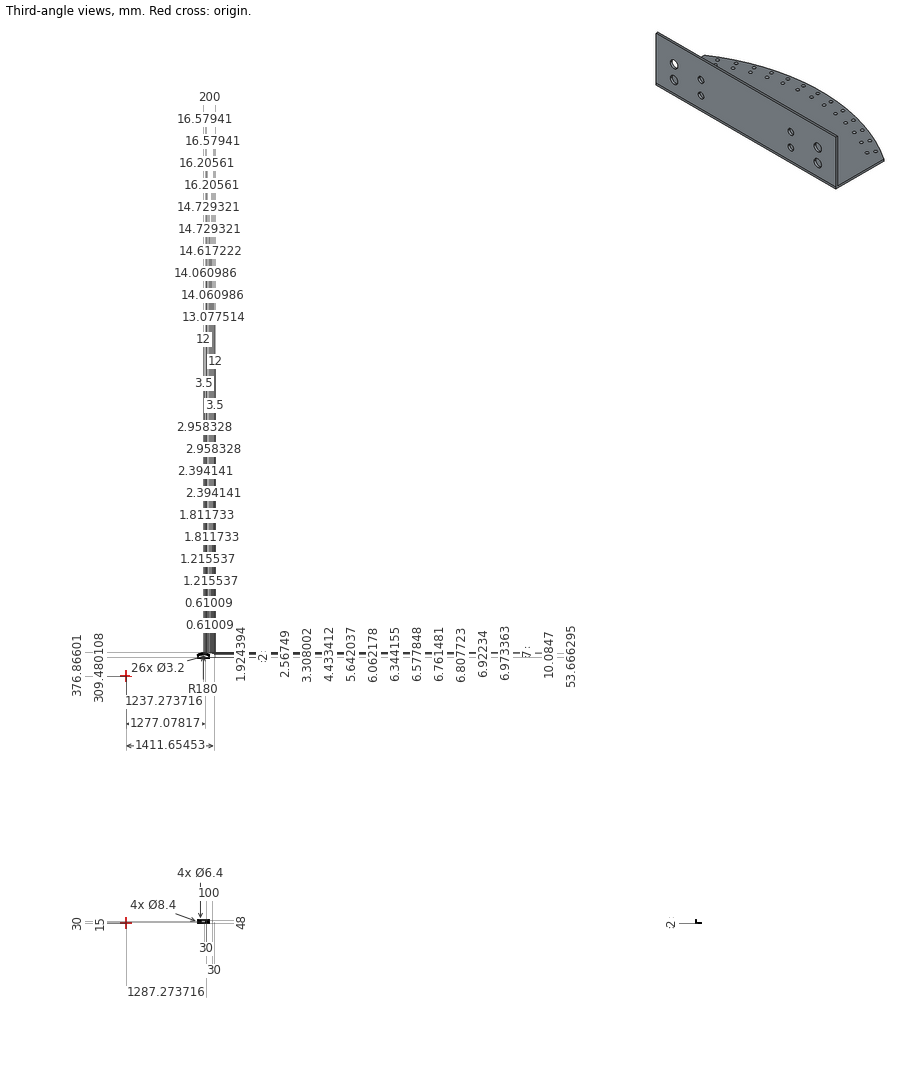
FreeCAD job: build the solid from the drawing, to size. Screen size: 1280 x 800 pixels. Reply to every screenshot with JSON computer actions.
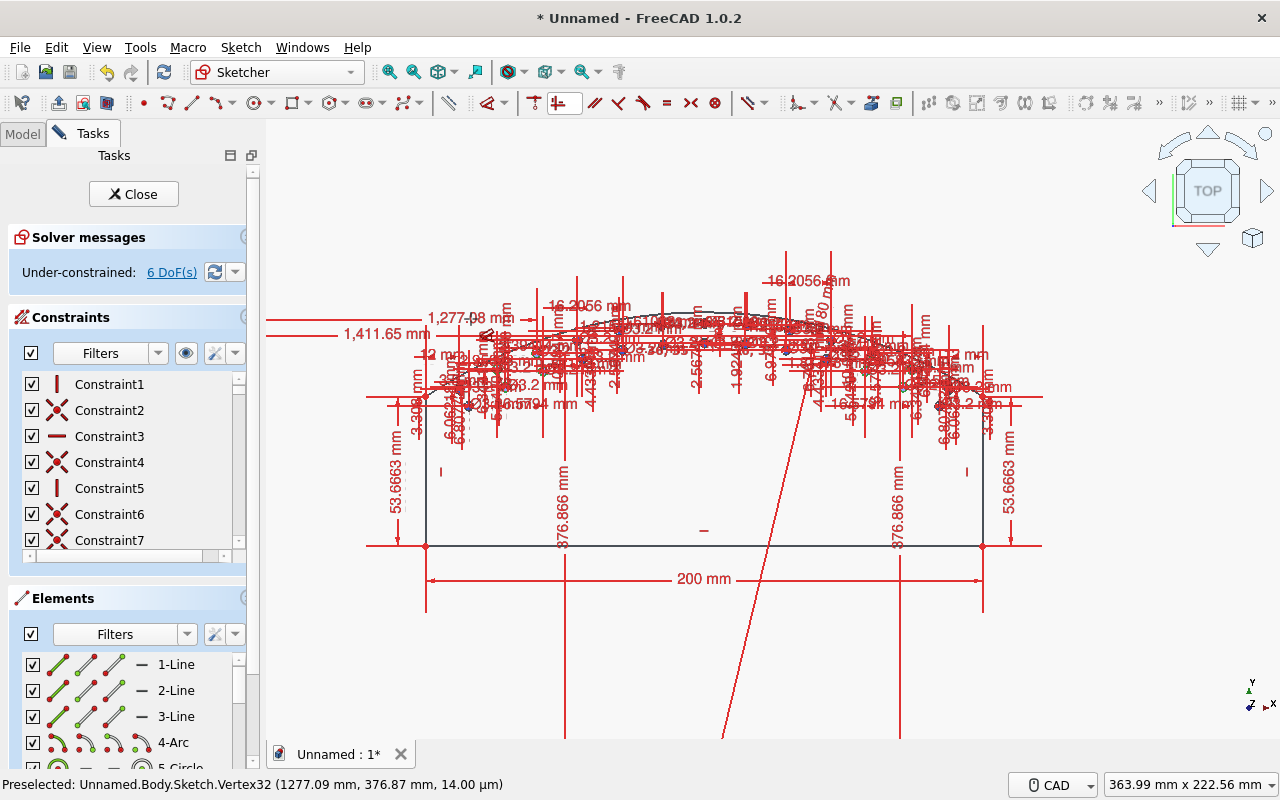
{"action": "left_click", "coordinate": [940, 406]}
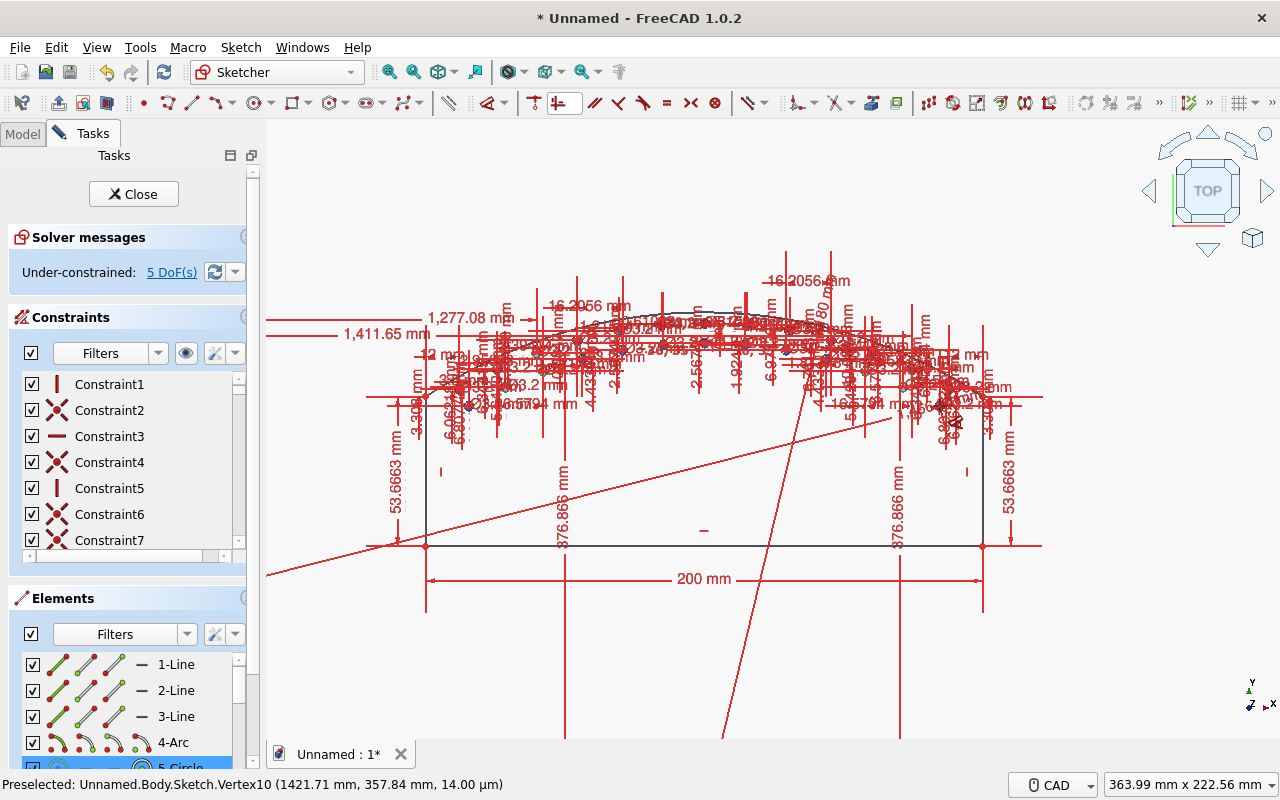
{"action": "left_click", "coordinate": [903, 387]}
{"action": "left_click", "coordinate": [922, 440]}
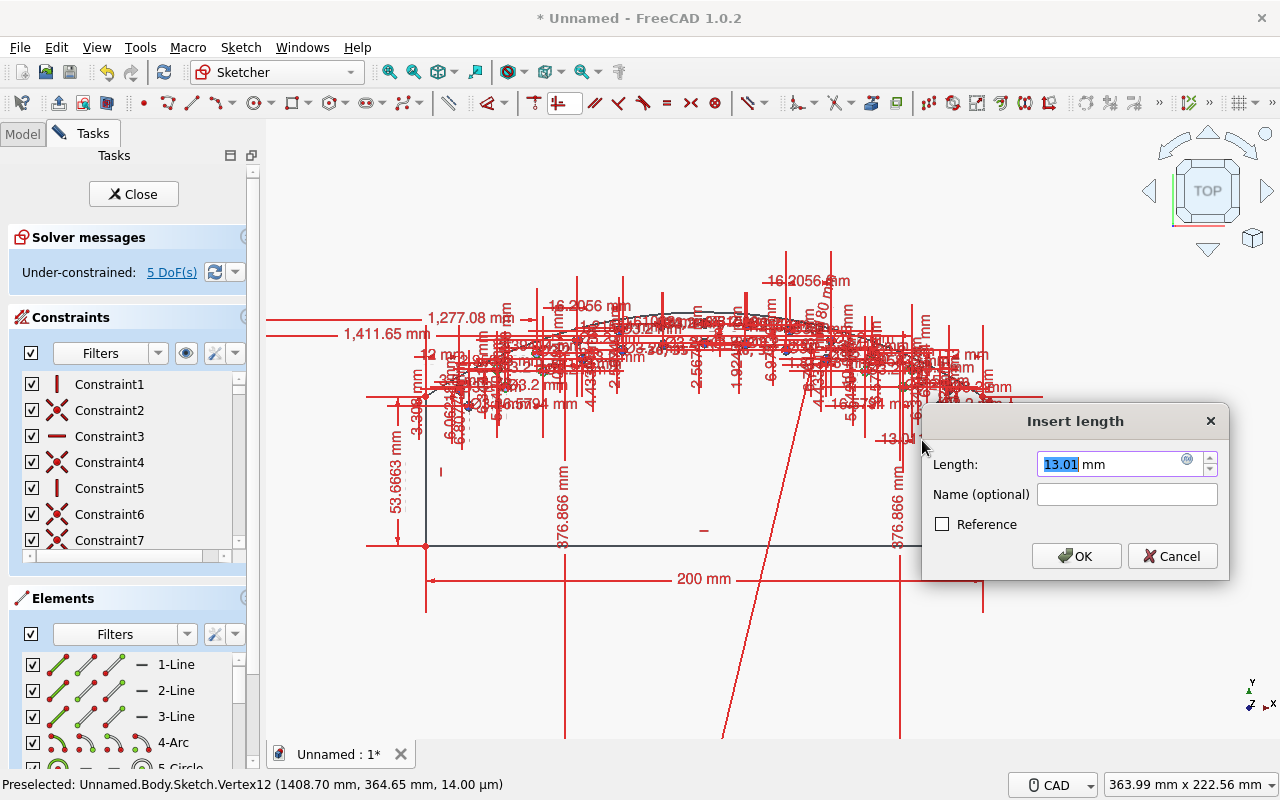
{"action": "type", "text": "13.077514"}
{"action": "key", "text": "Return"}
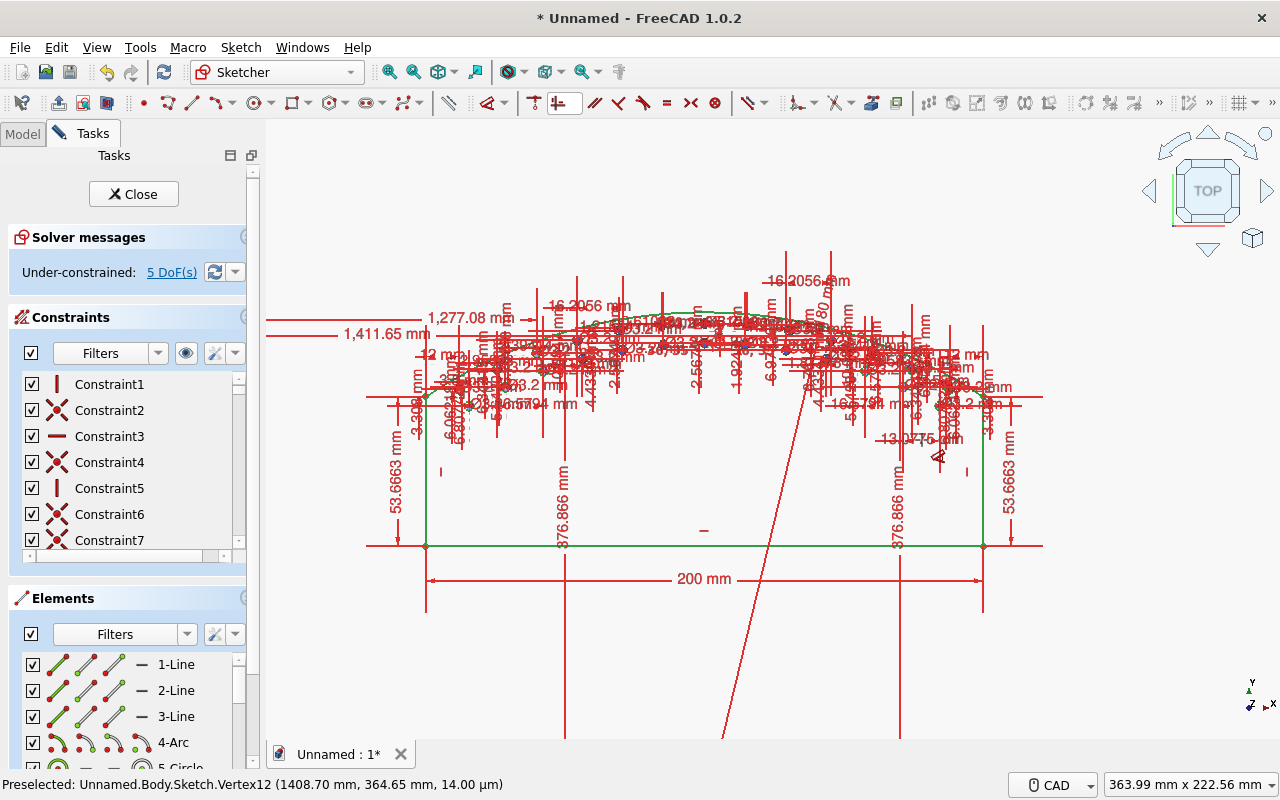
{"action": "left_click", "coordinate": [865, 371]}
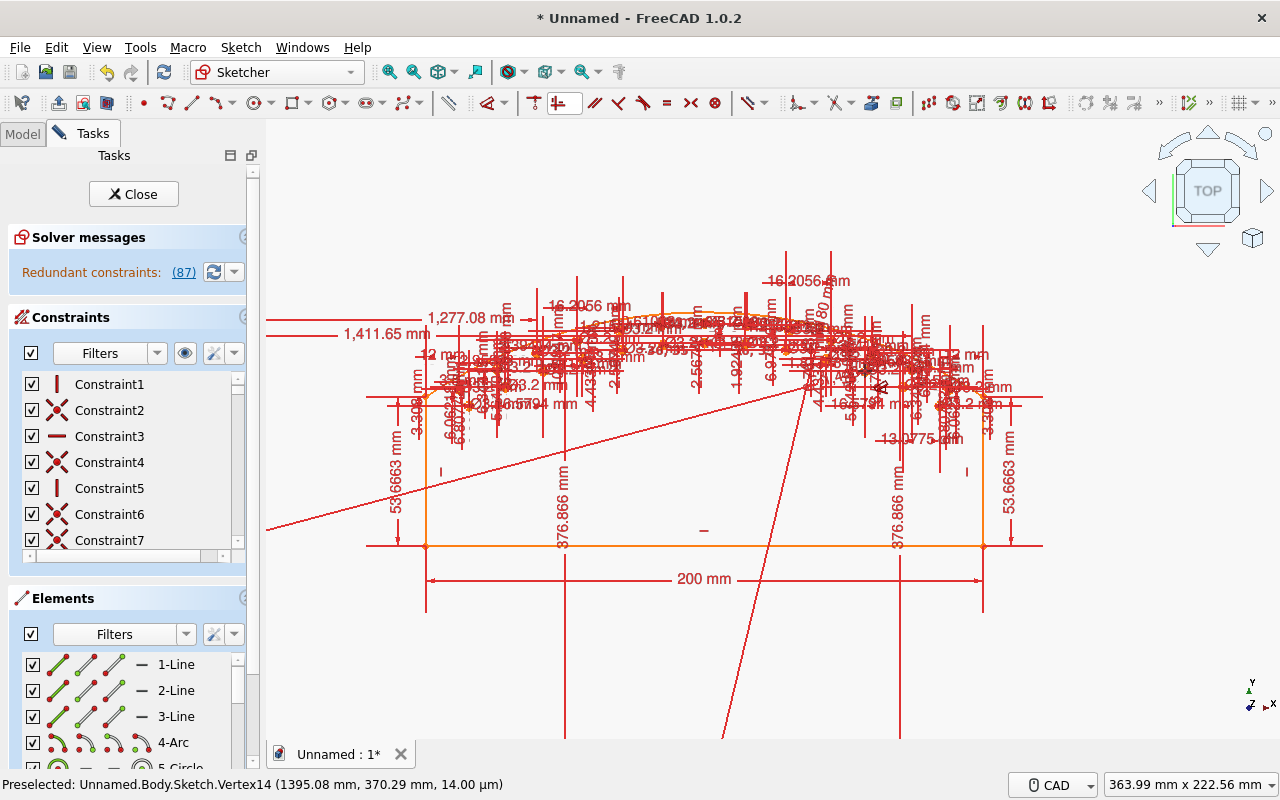
{"action": "left_click", "coordinate": [826, 359]}
{"action": "left_click", "coordinate": [846, 429]}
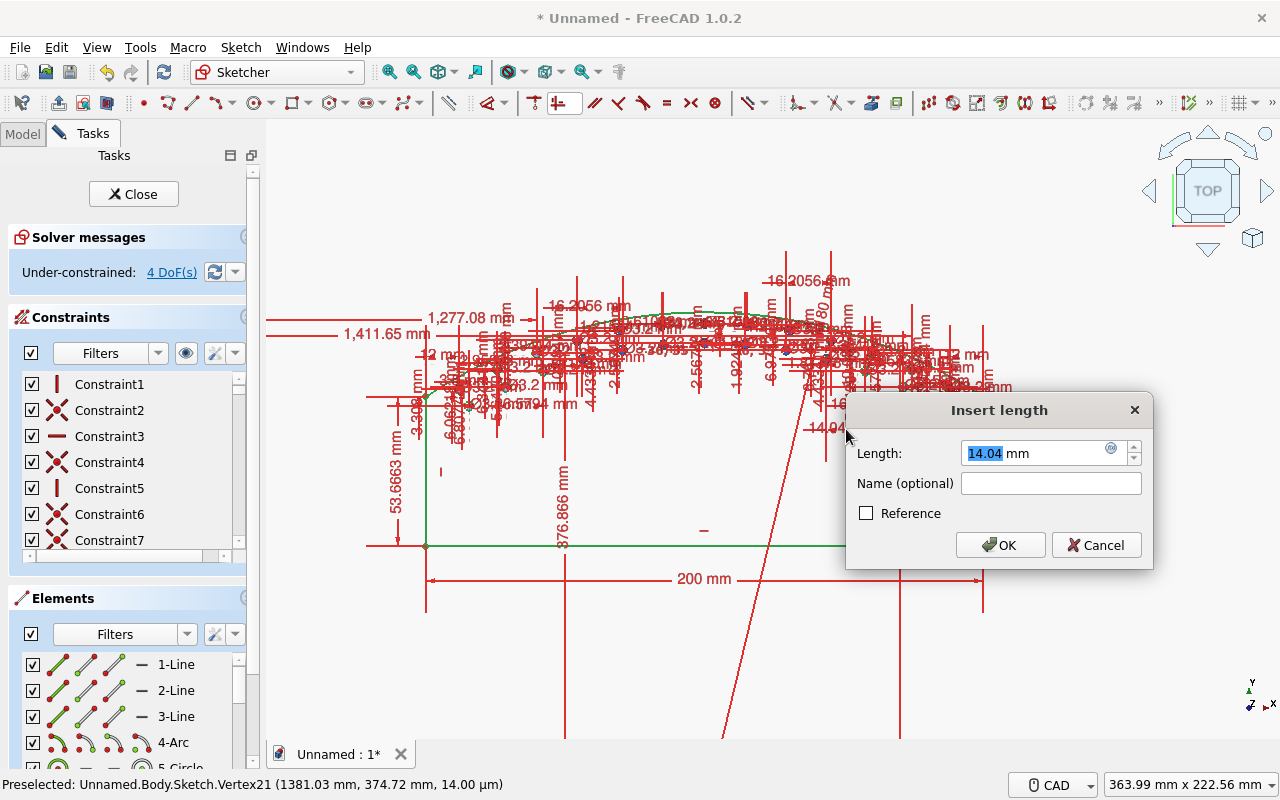
{"action": "type", "text": "14.060986"}
{"action": "key", "text": "Return"}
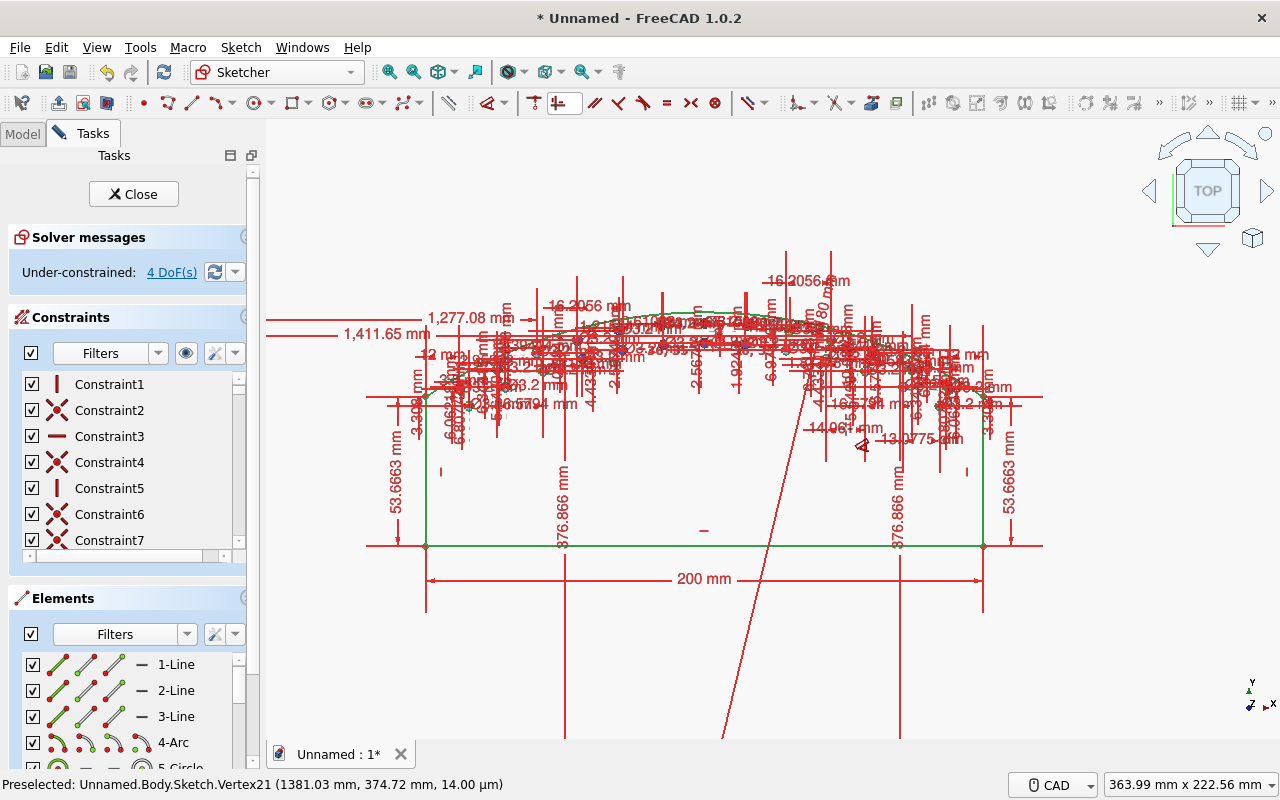
{"action": "left_click", "coordinate": [786, 350]}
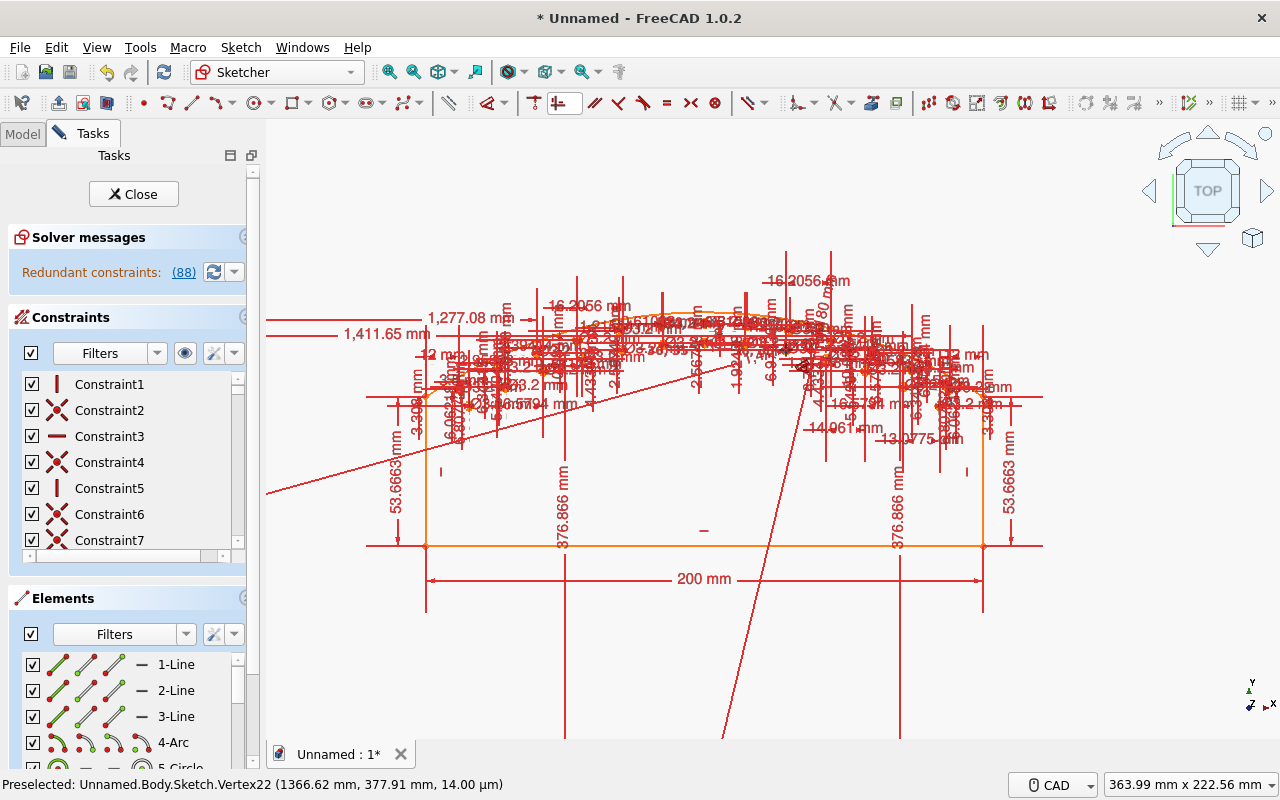
{"action": "left_click", "coordinate": [745, 345]}
{"action": "left_click", "coordinate": [766, 408]}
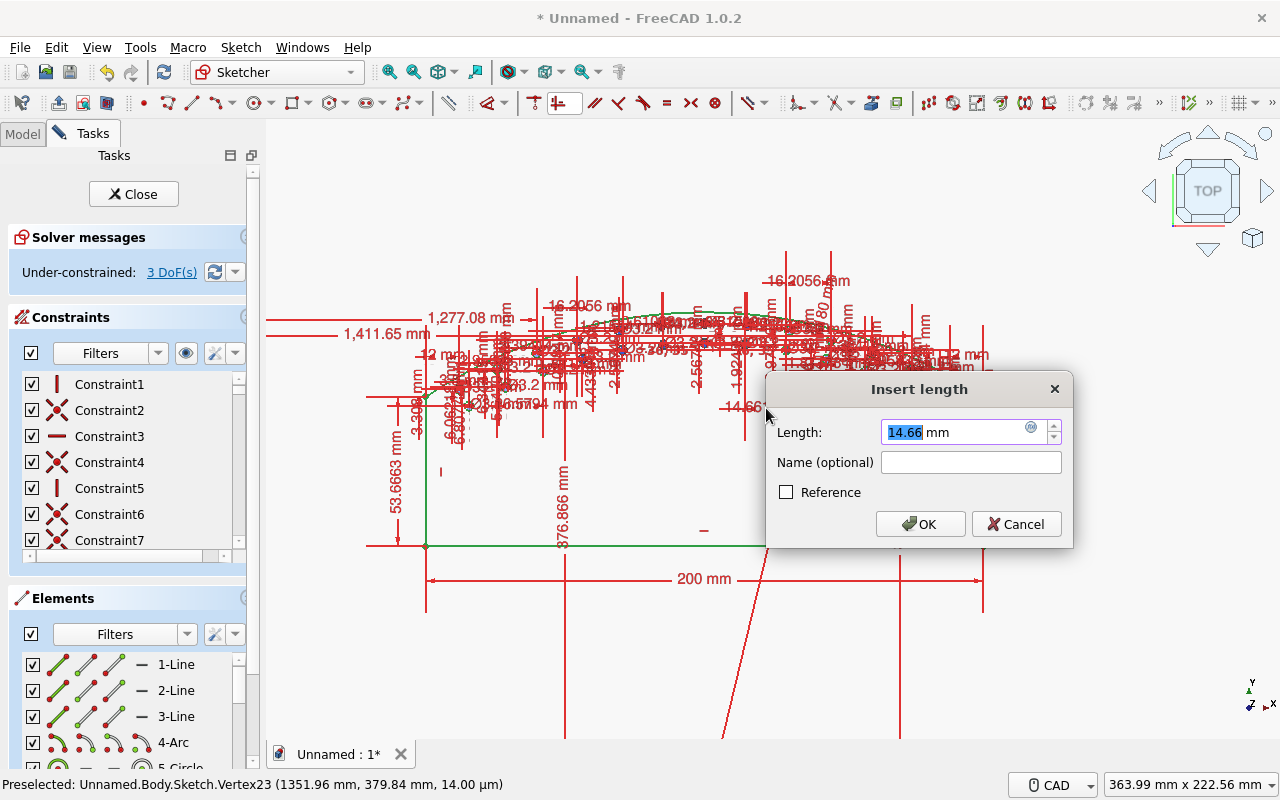
{"action": "type", "text": "14.617222"}
{"action": "key", "text": "Return"}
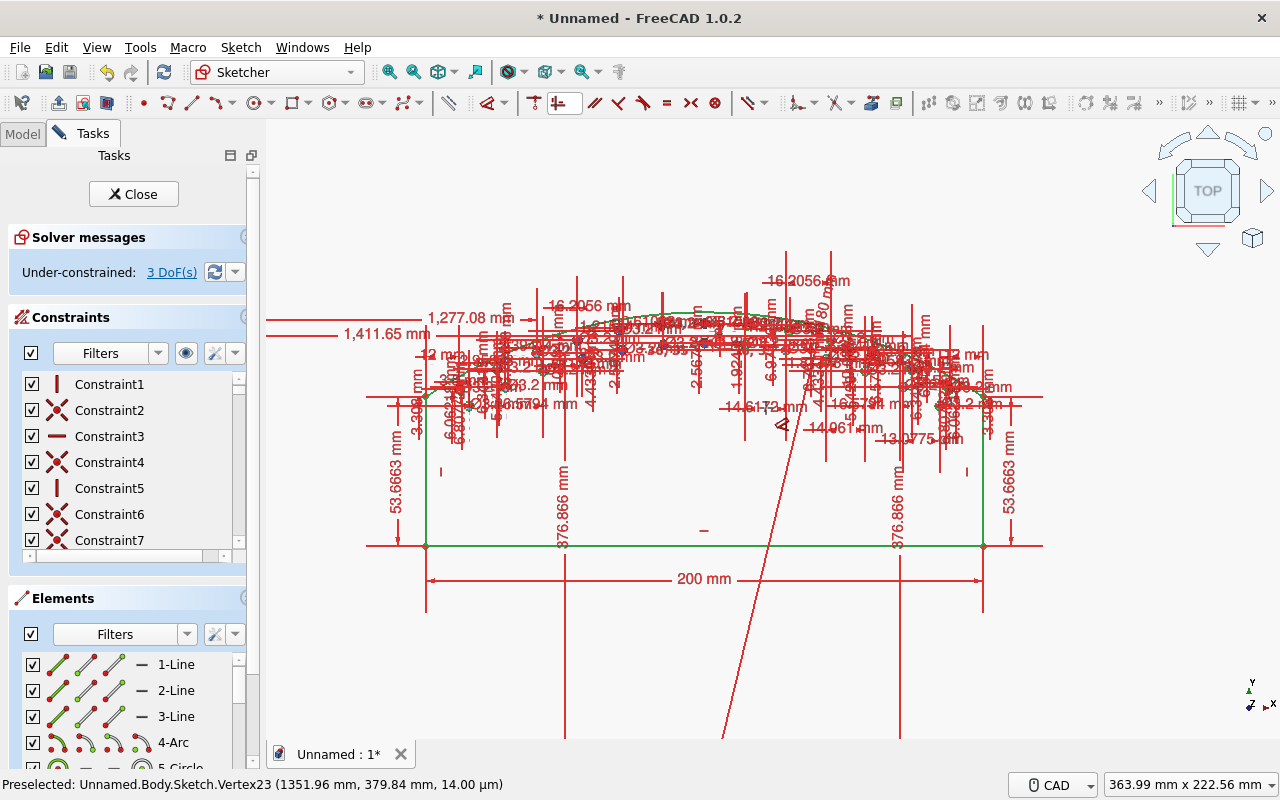
{"action": "left_click", "coordinate": [745, 345]}